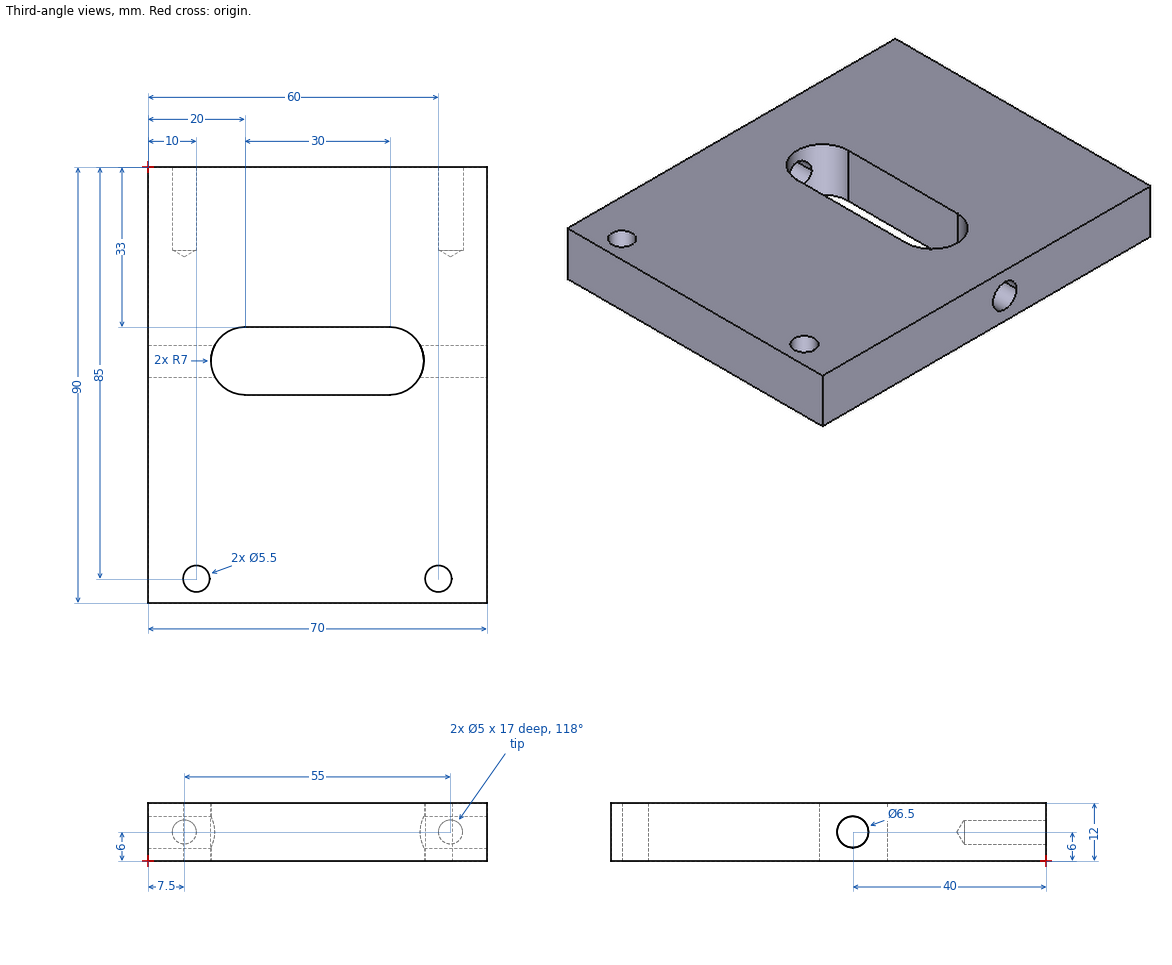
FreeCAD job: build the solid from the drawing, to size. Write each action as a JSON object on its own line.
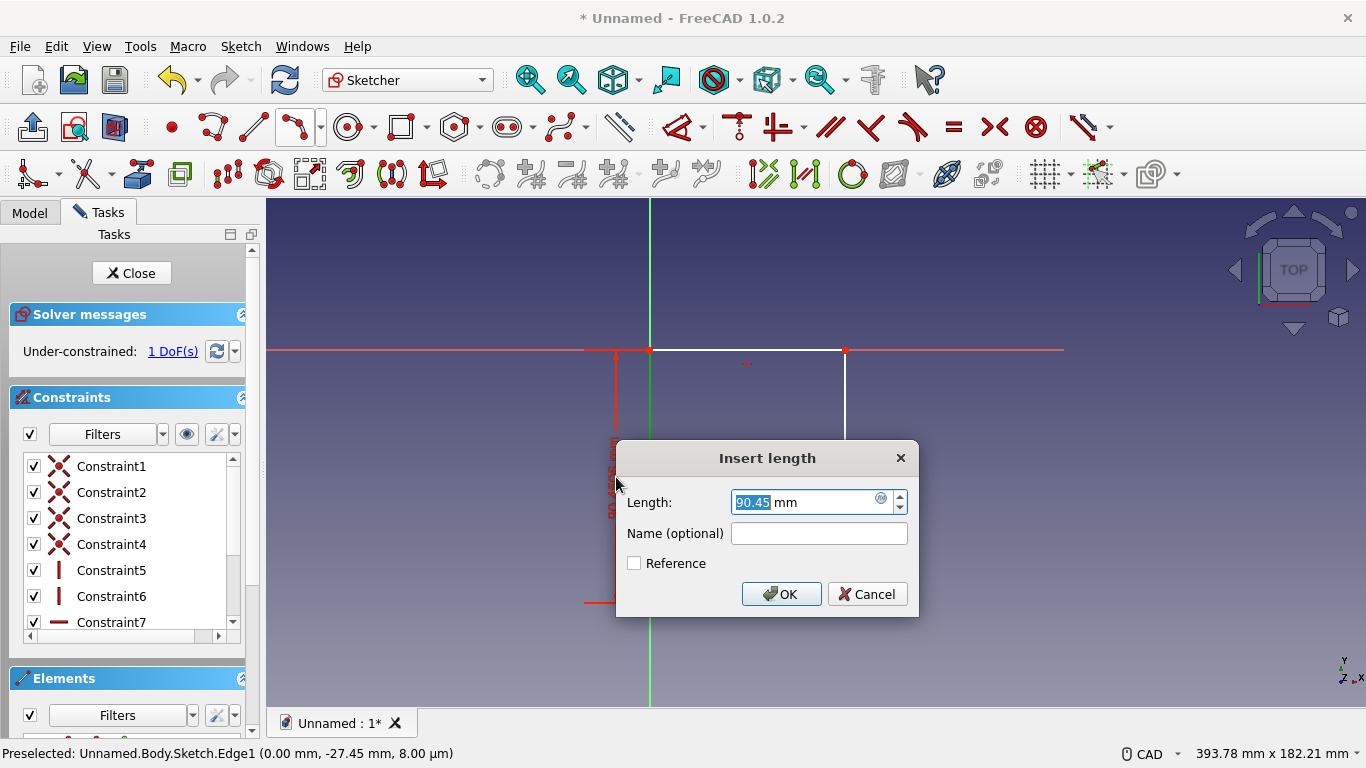
{"action": "type", "text": "90"}
{"action": "key", "text": "Return"}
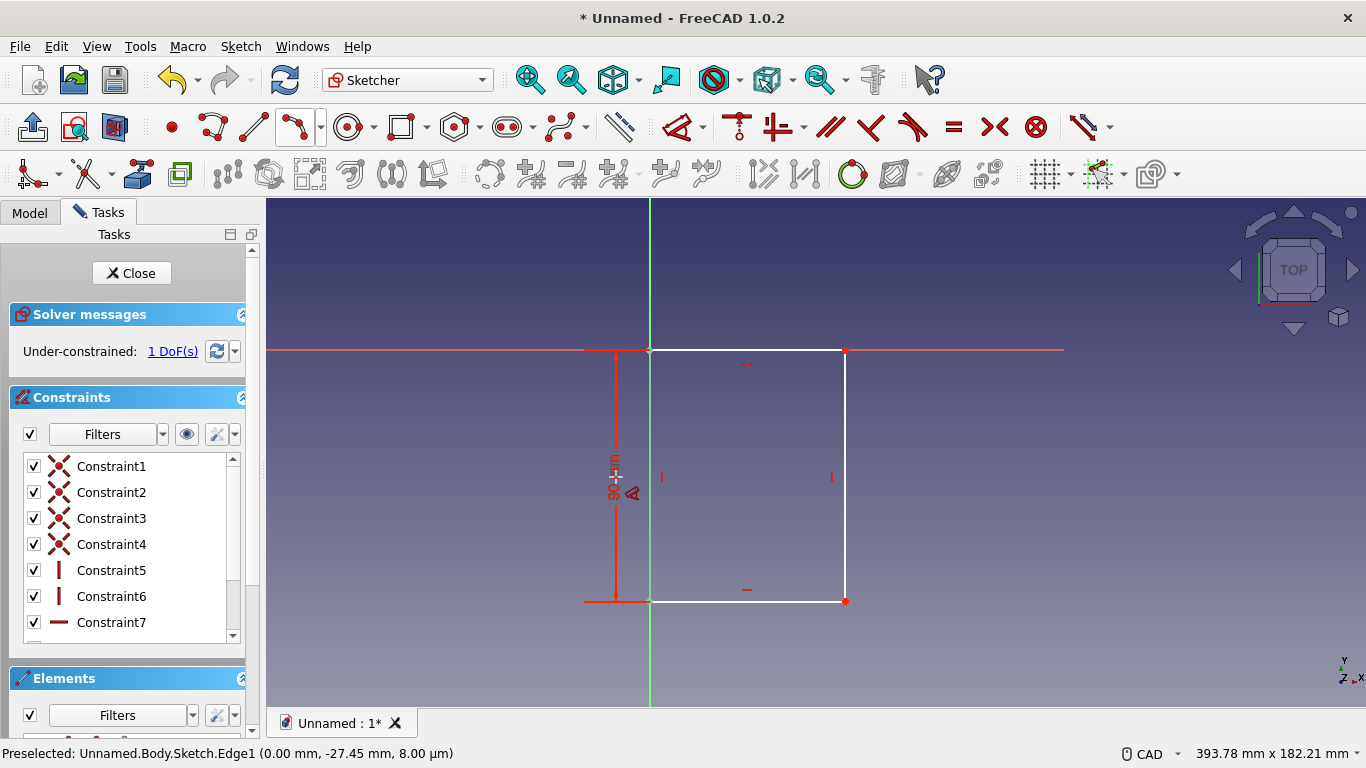
{"action": "left_click", "coordinate": [708, 602]}
{"action": "left_click", "coordinate": [747, 636]}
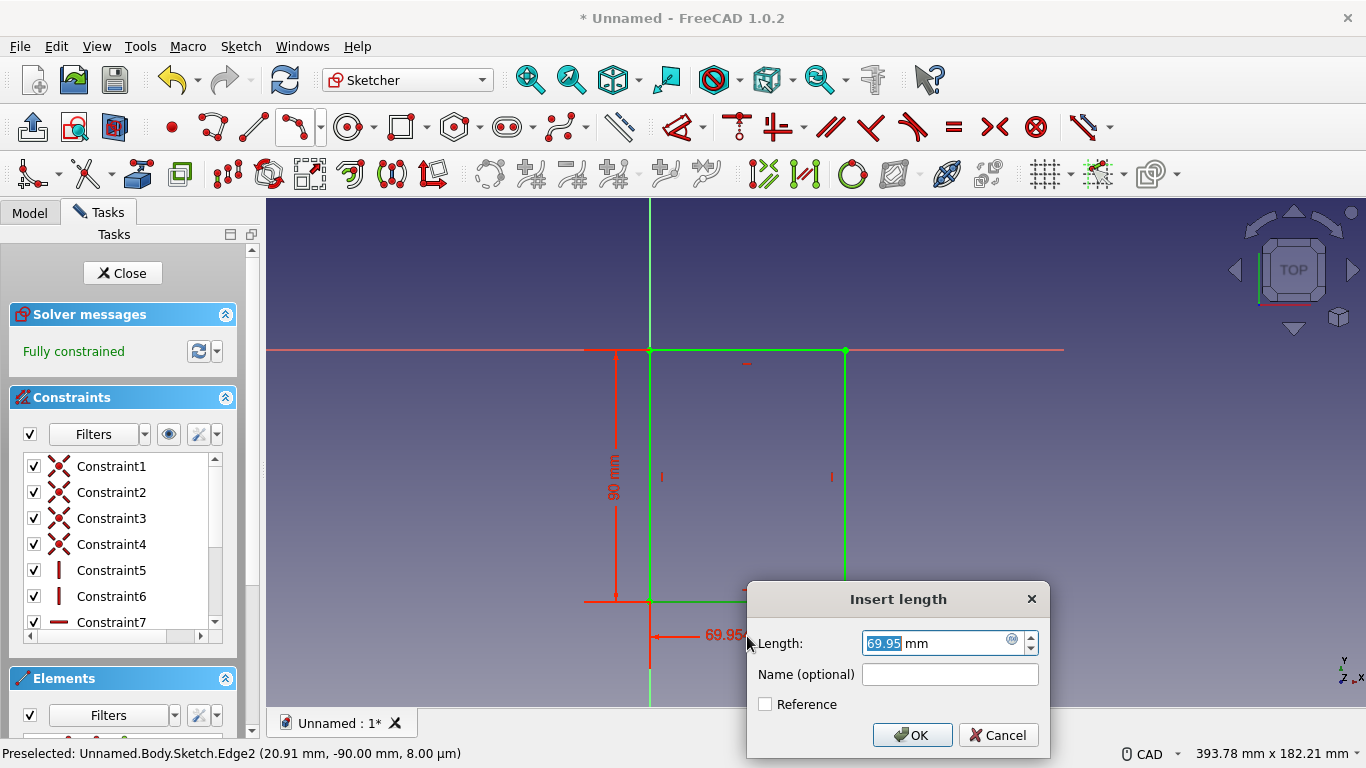
{"action": "type", "text": "70"}
{"action": "key", "text": "Return"}
{"action": "key", "text": "Escape"}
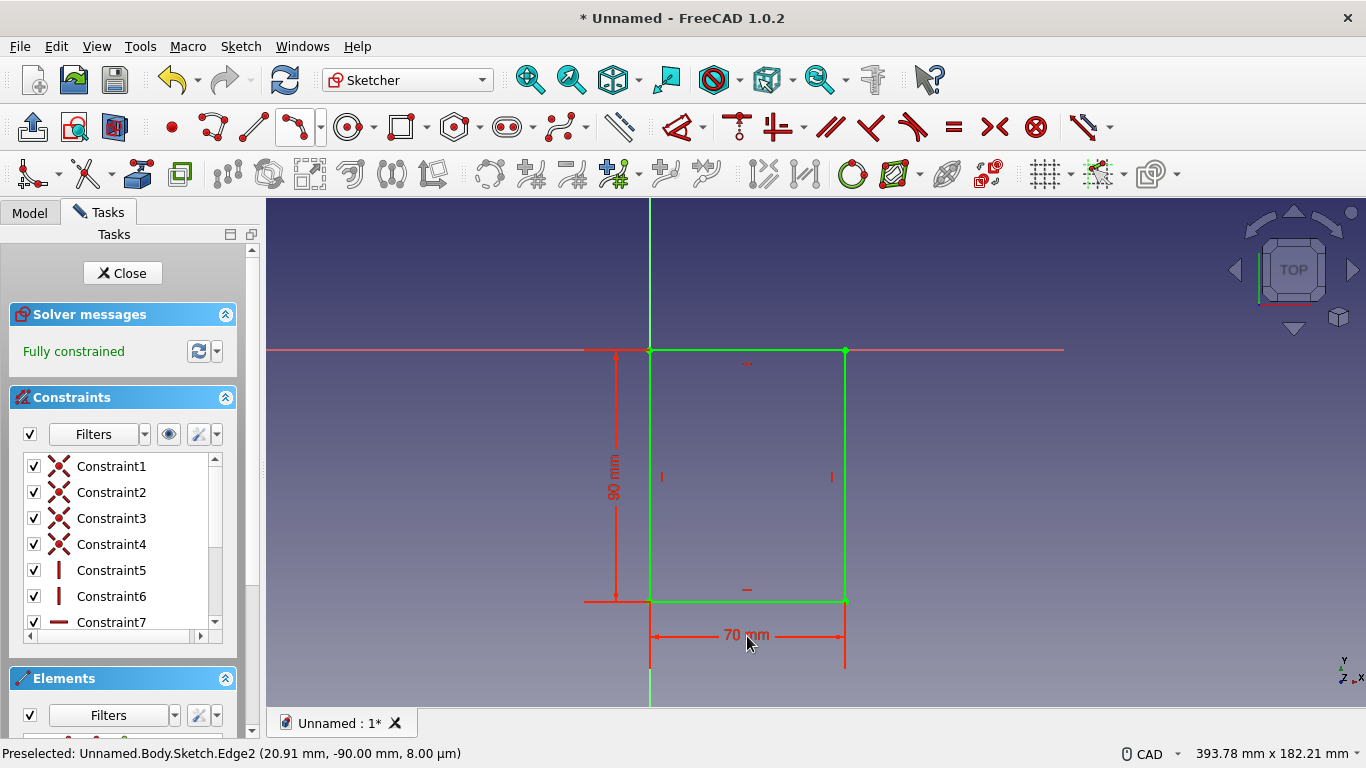
{"action": "left_click", "coordinate": [123, 273]}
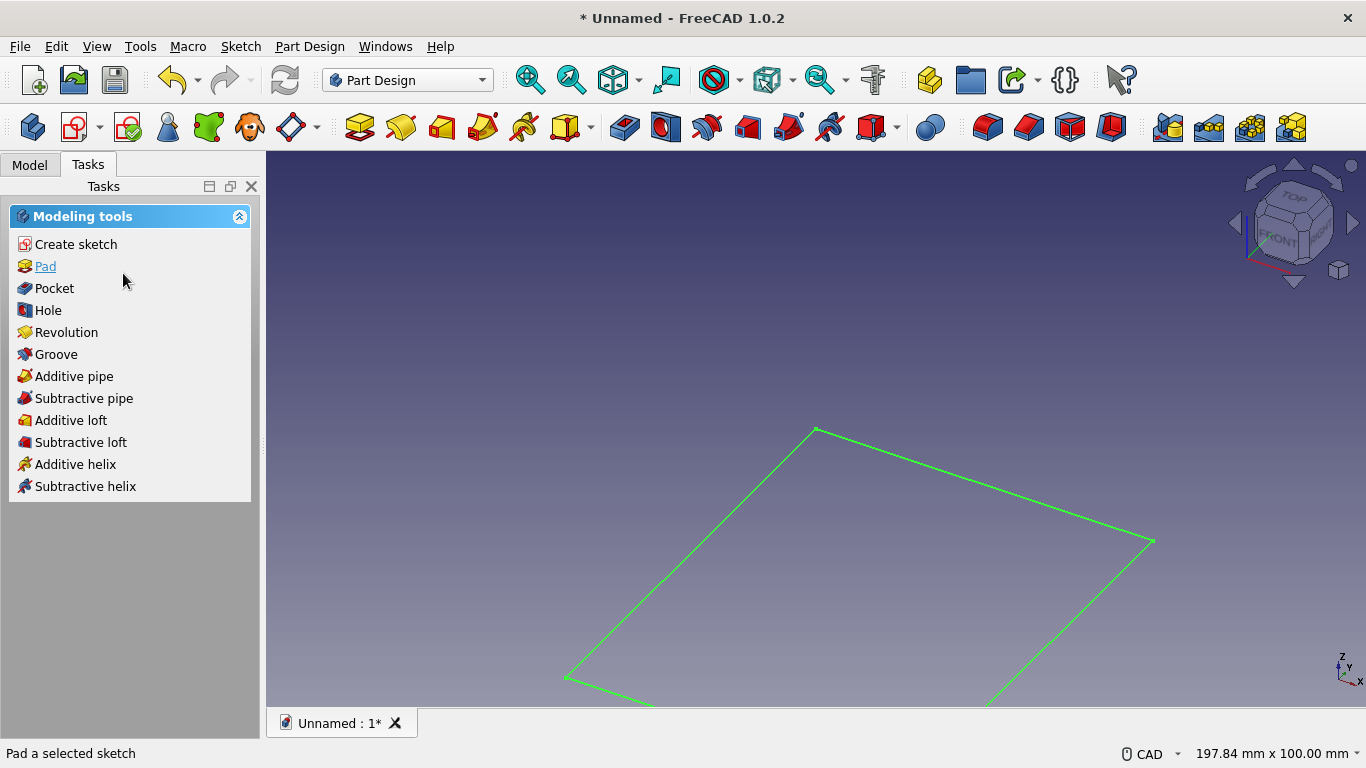
{"action": "left_click", "coordinate": [360, 128]}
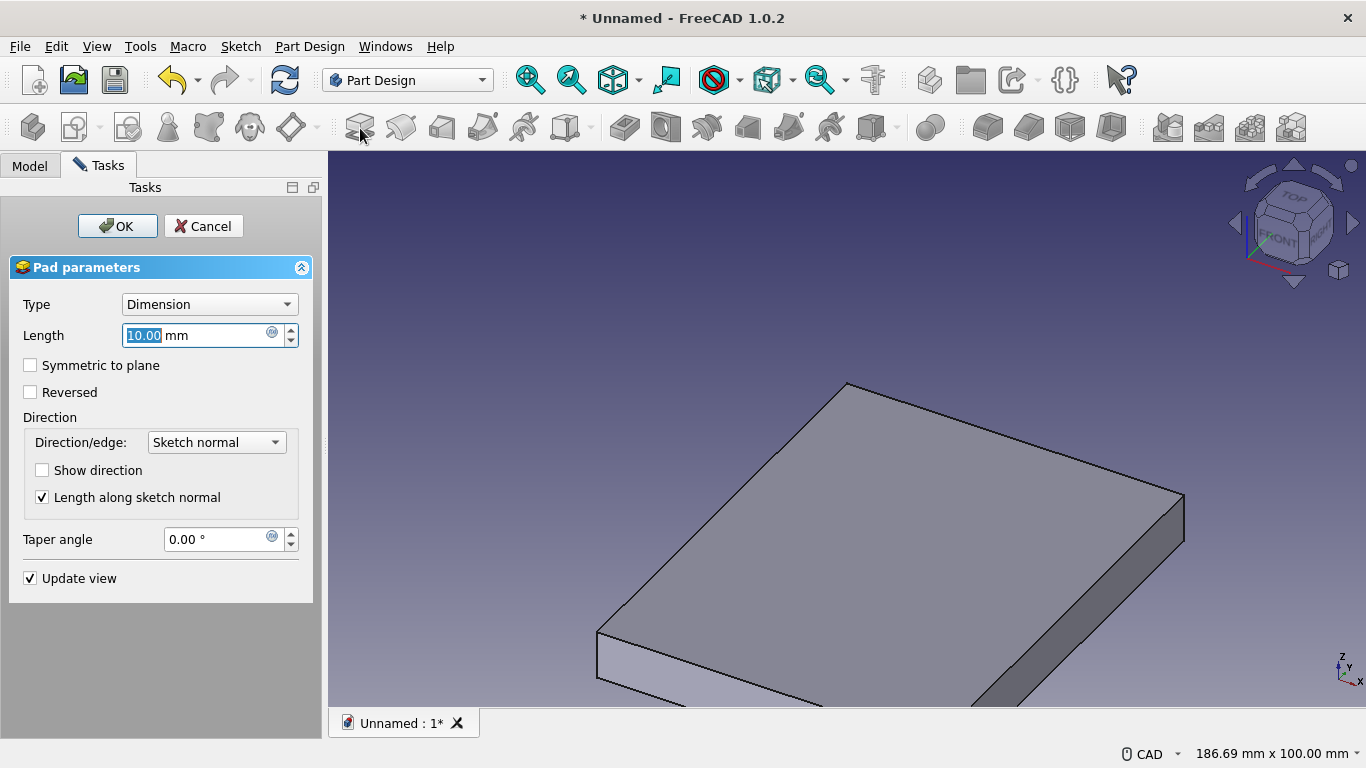
{"action": "type", "text": "12"}
{"action": "key", "text": "Tab"}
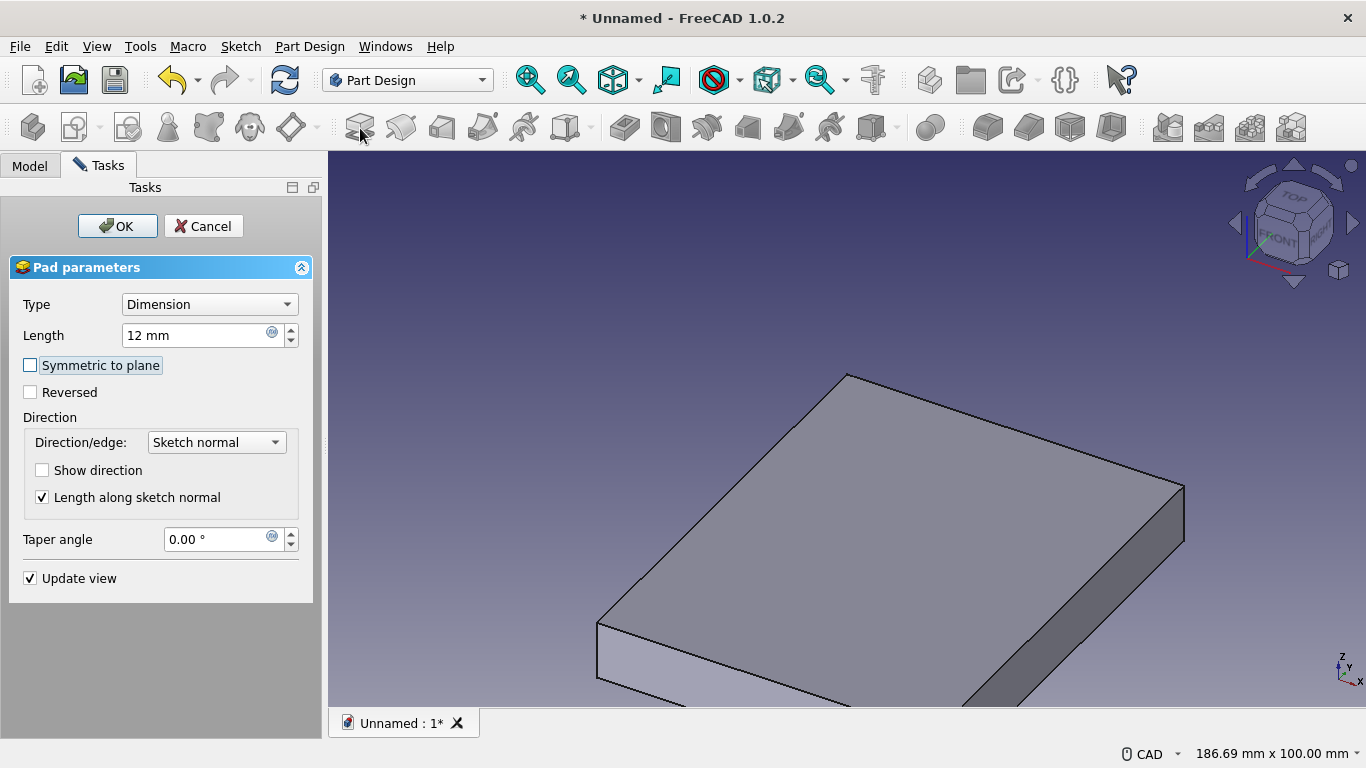
{"action": "left_click", "coordinate": [118, 226]}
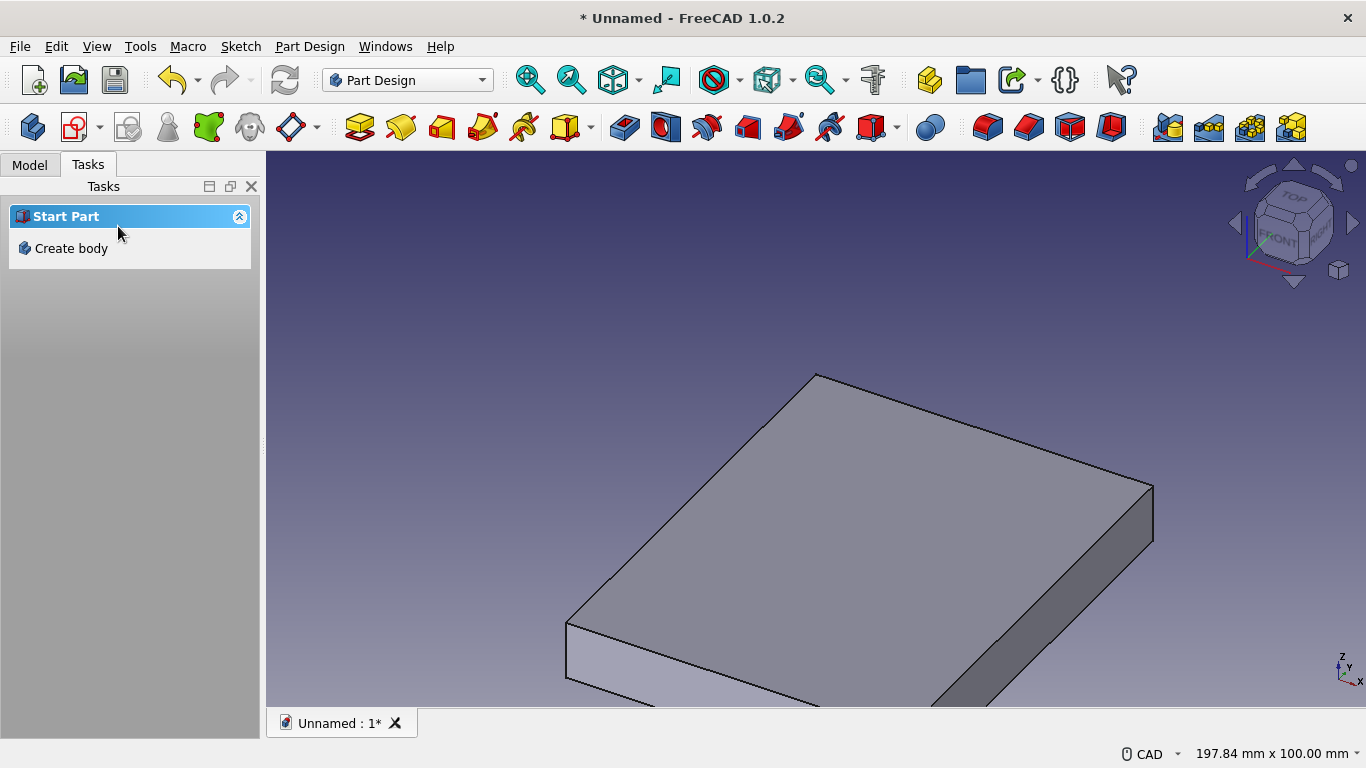
{"action": "left_click", "coordinate": [531, 80]}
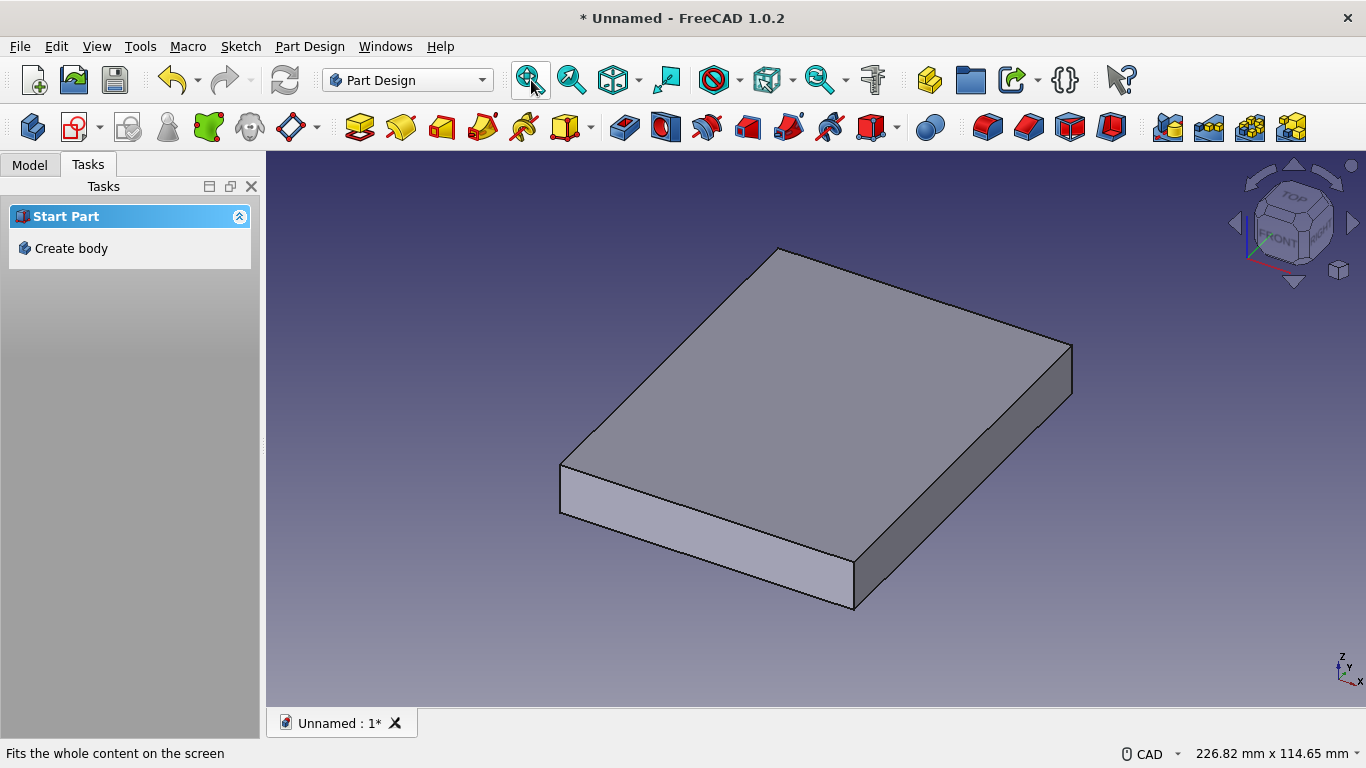
{"action": "left_click", "coordinate": [816, 404]}